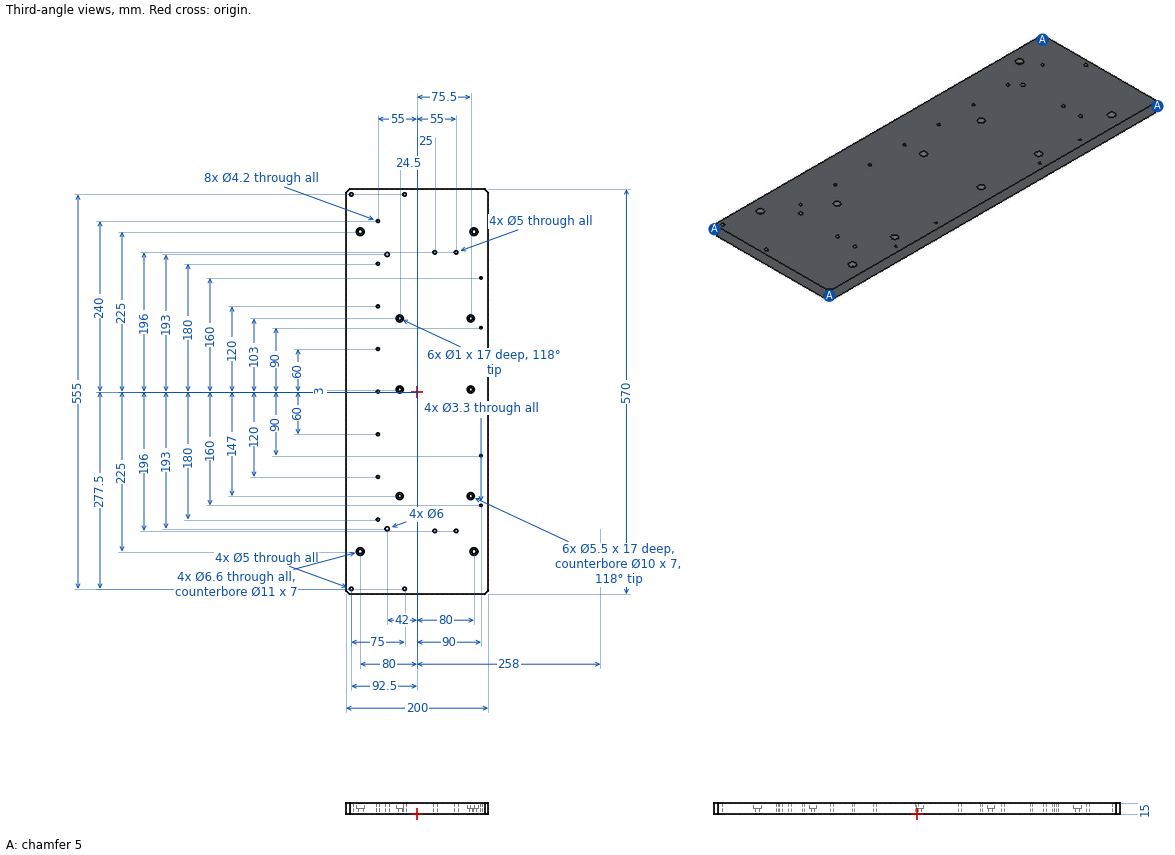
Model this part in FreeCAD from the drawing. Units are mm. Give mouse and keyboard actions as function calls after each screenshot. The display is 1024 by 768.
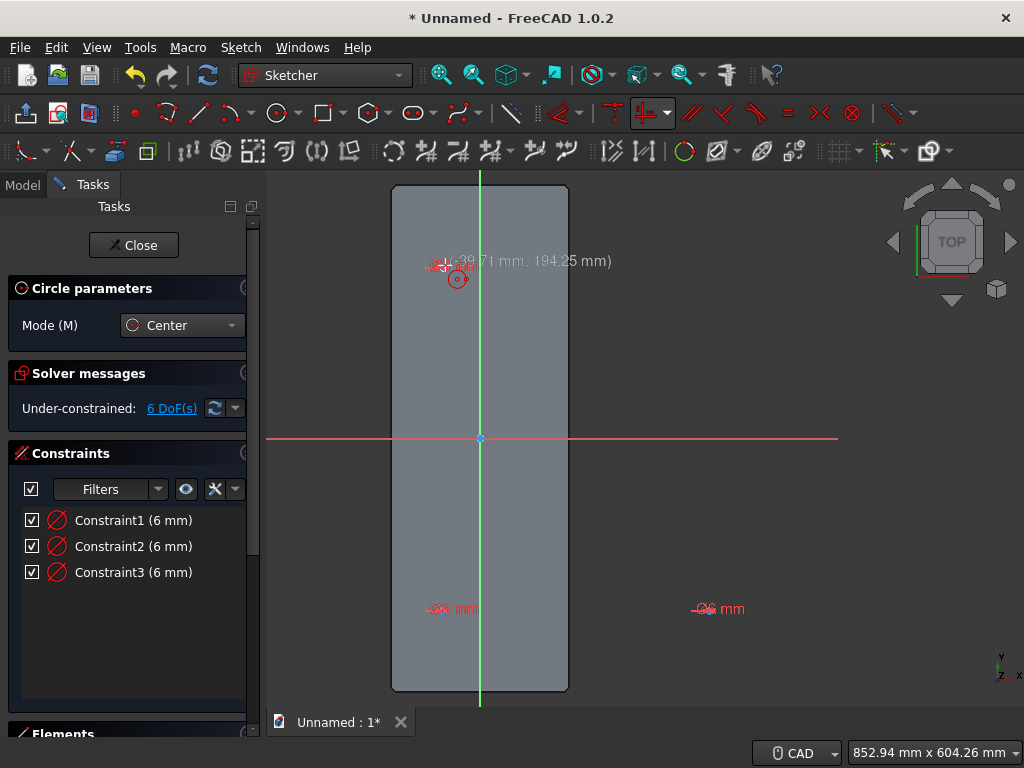
scroll(710, 267, up, 11)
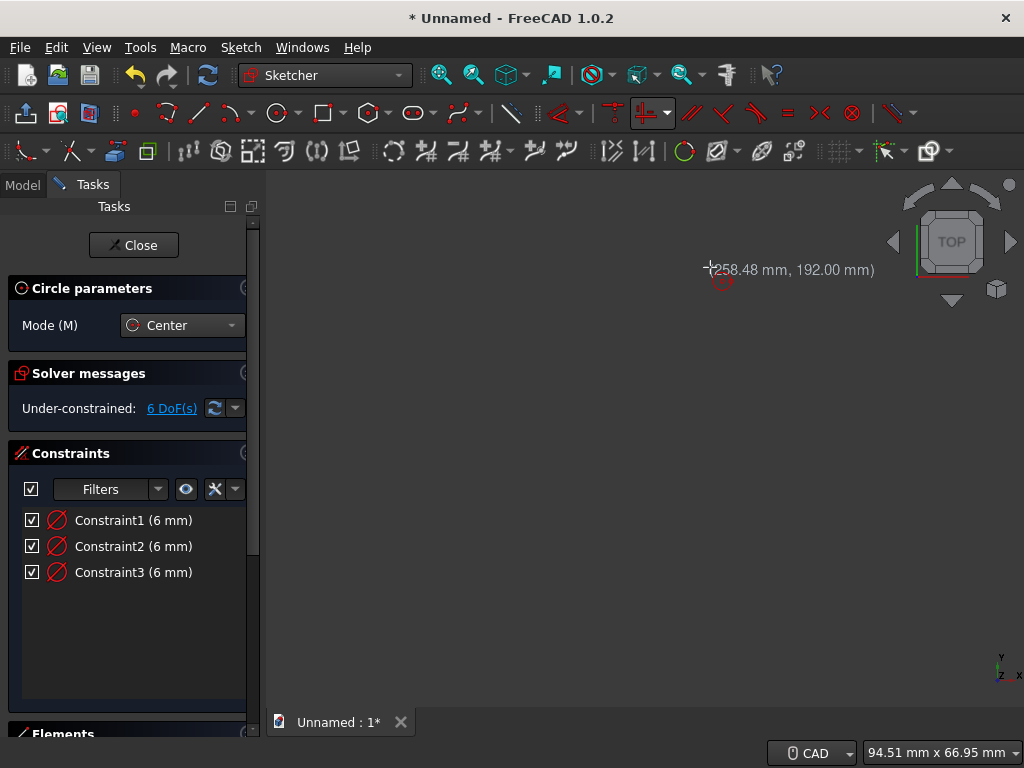
scroll(711, 267, down, 11)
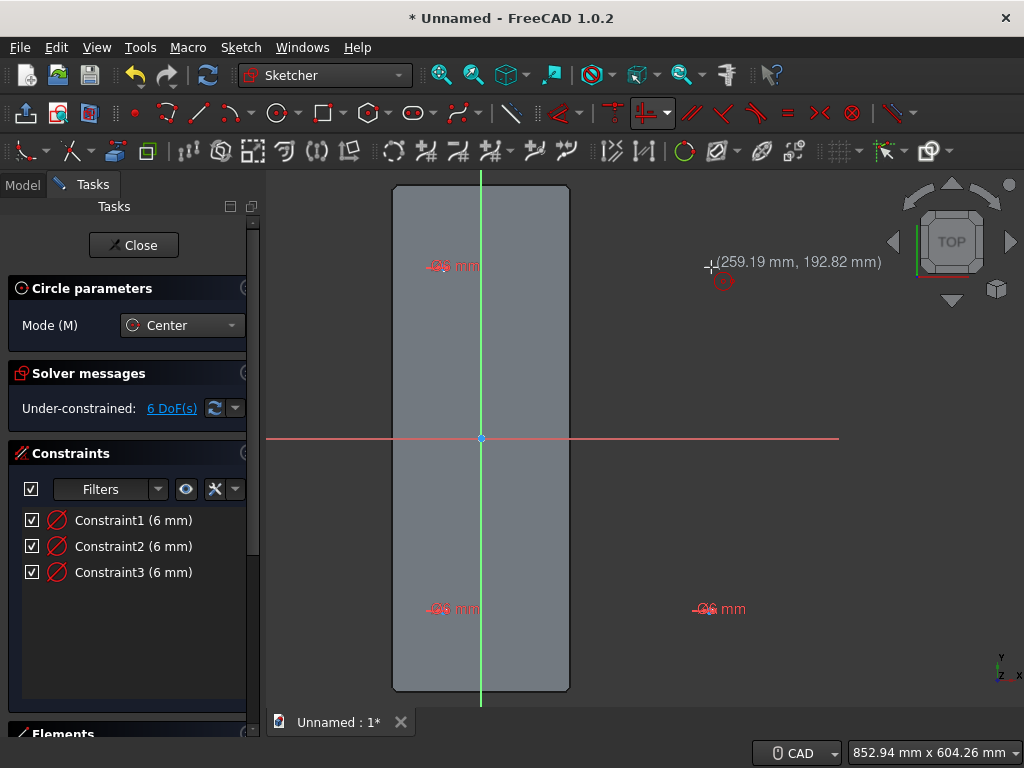
click(710, 267)
move(712, 265)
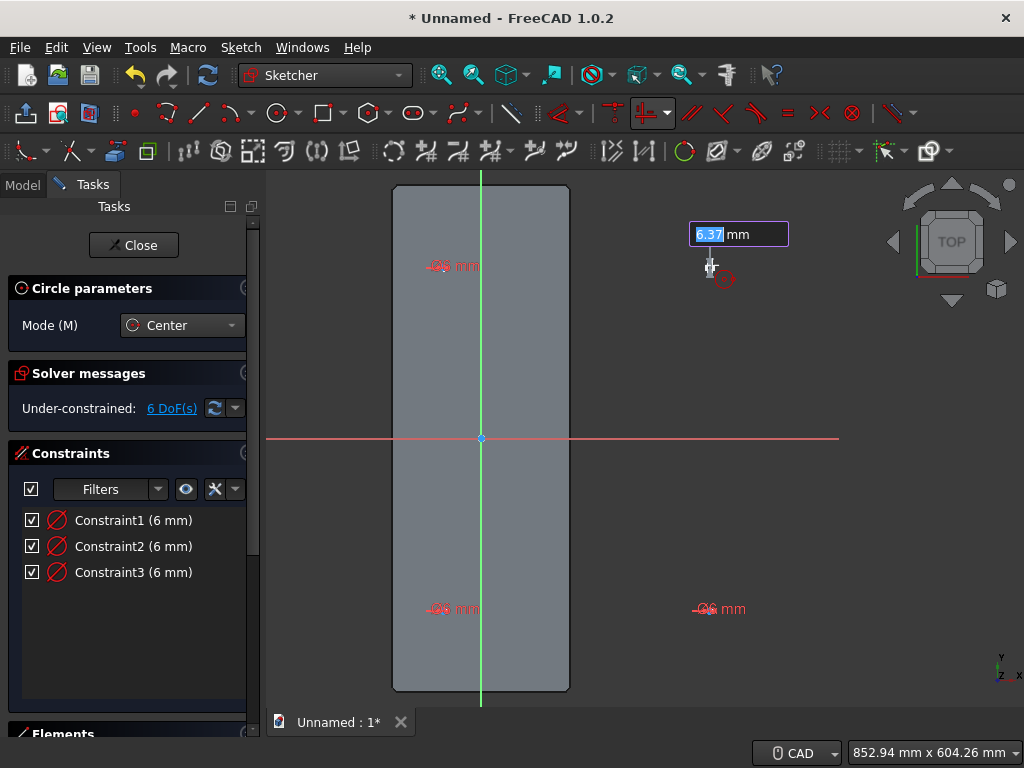
text(6)
key(Return)
key(Escape)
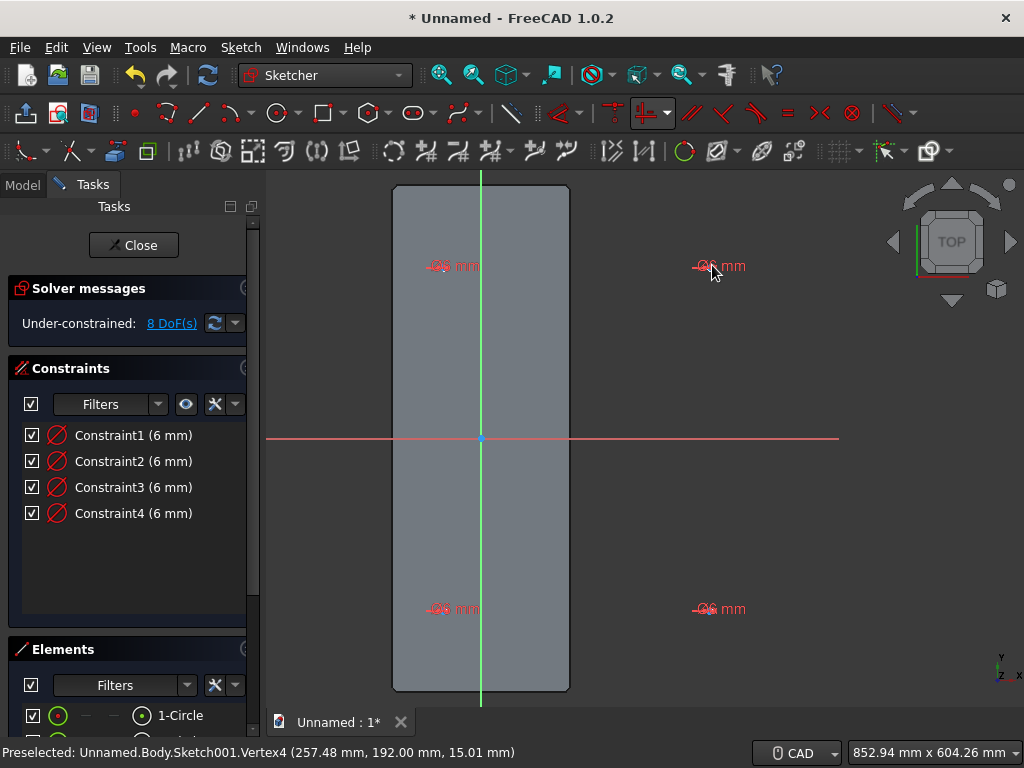
click(444, 611)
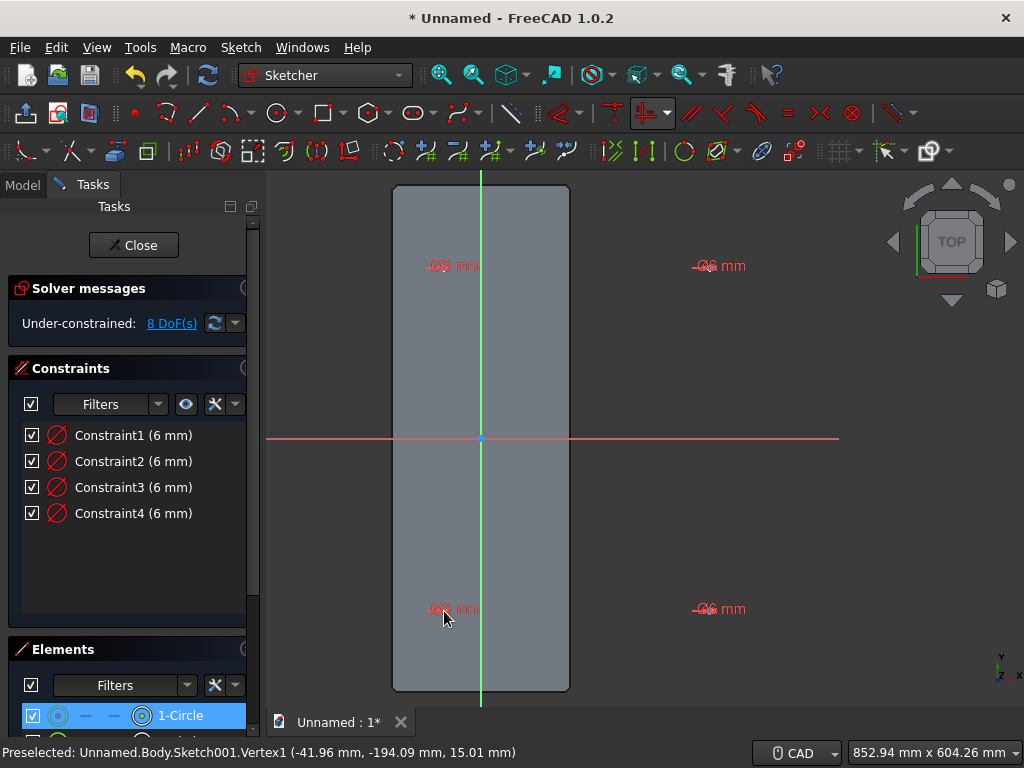
click(710, 611)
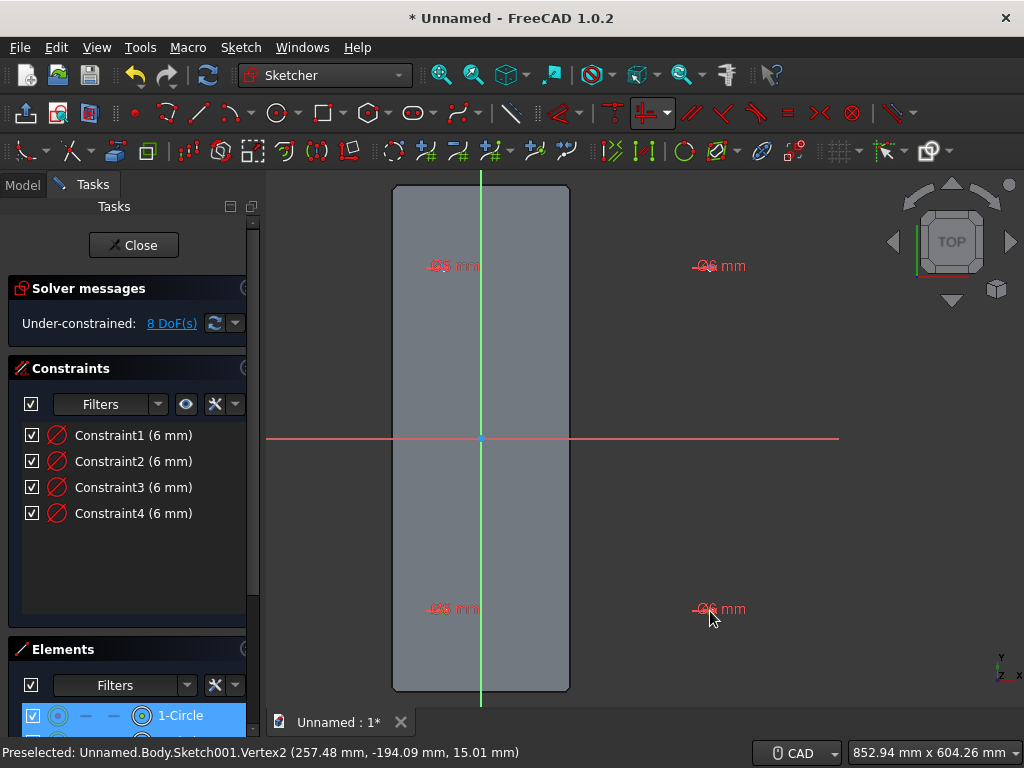
click(670, 114)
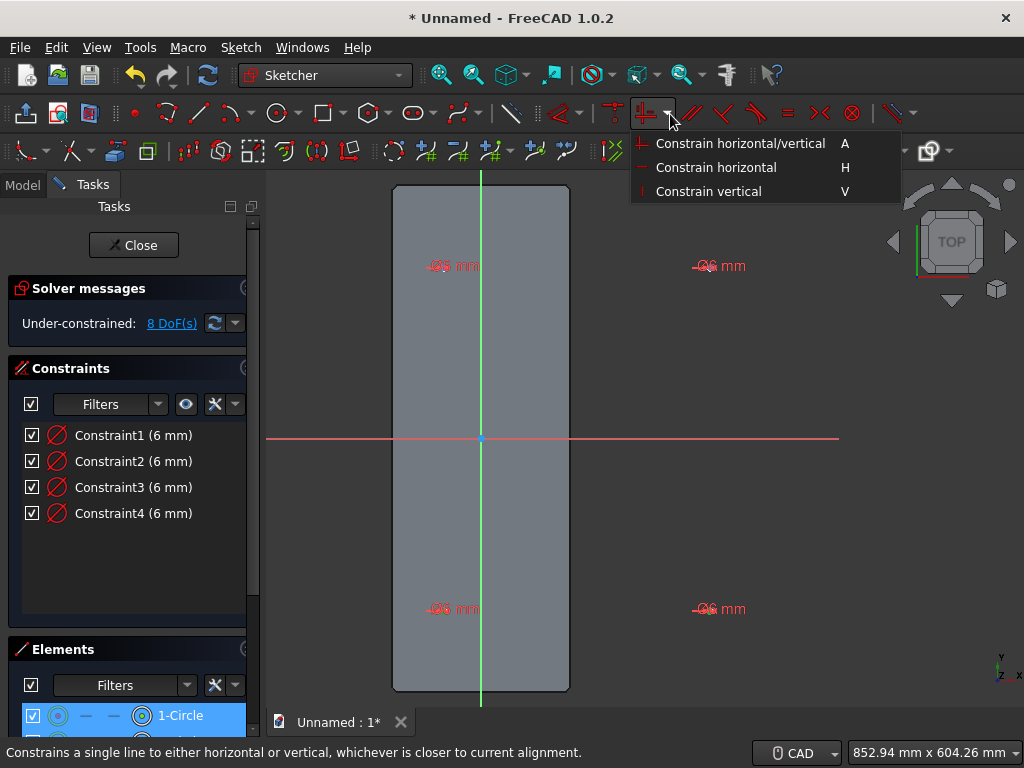
click(766, 167)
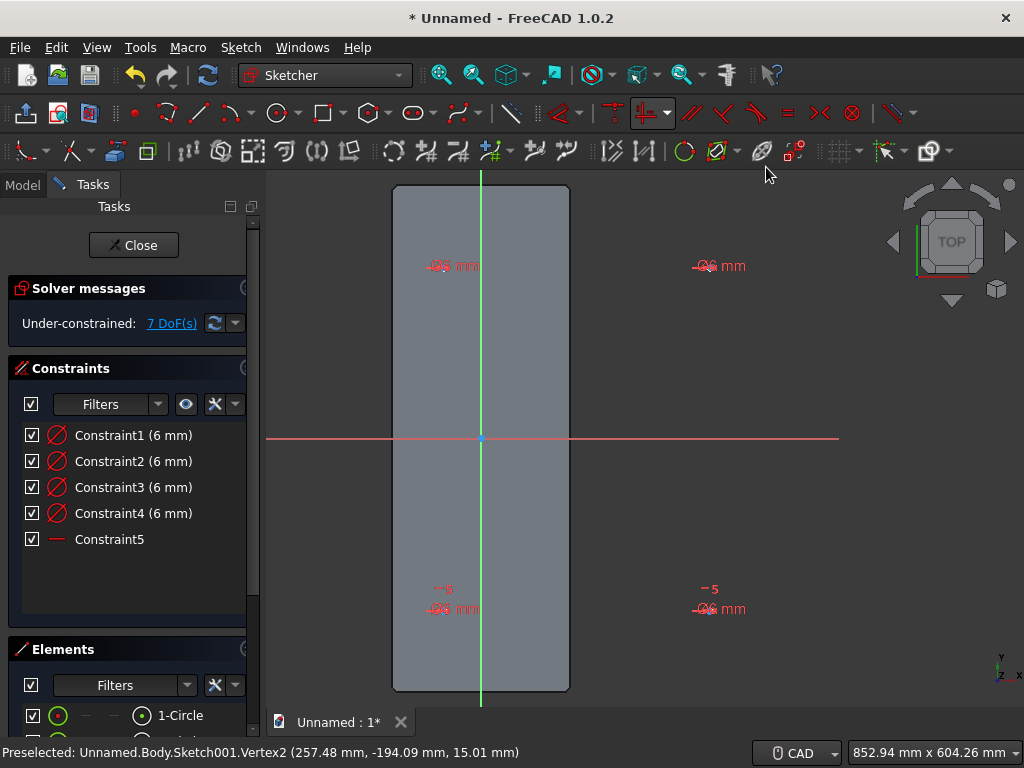
click(444, 611)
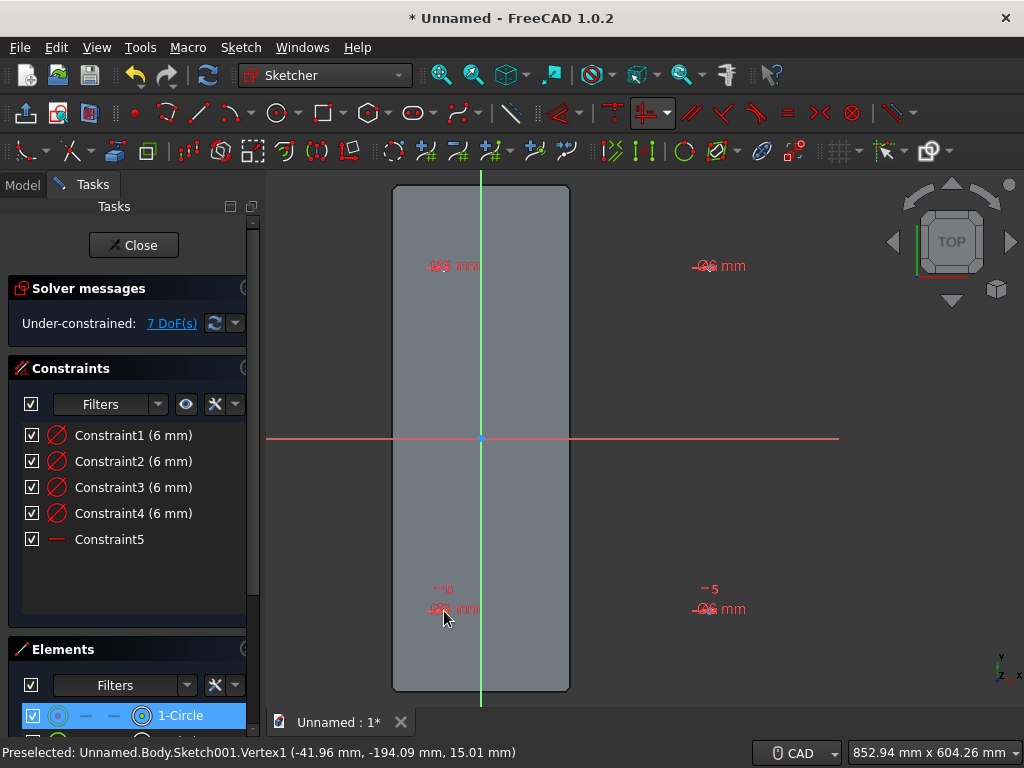
click(444, 268)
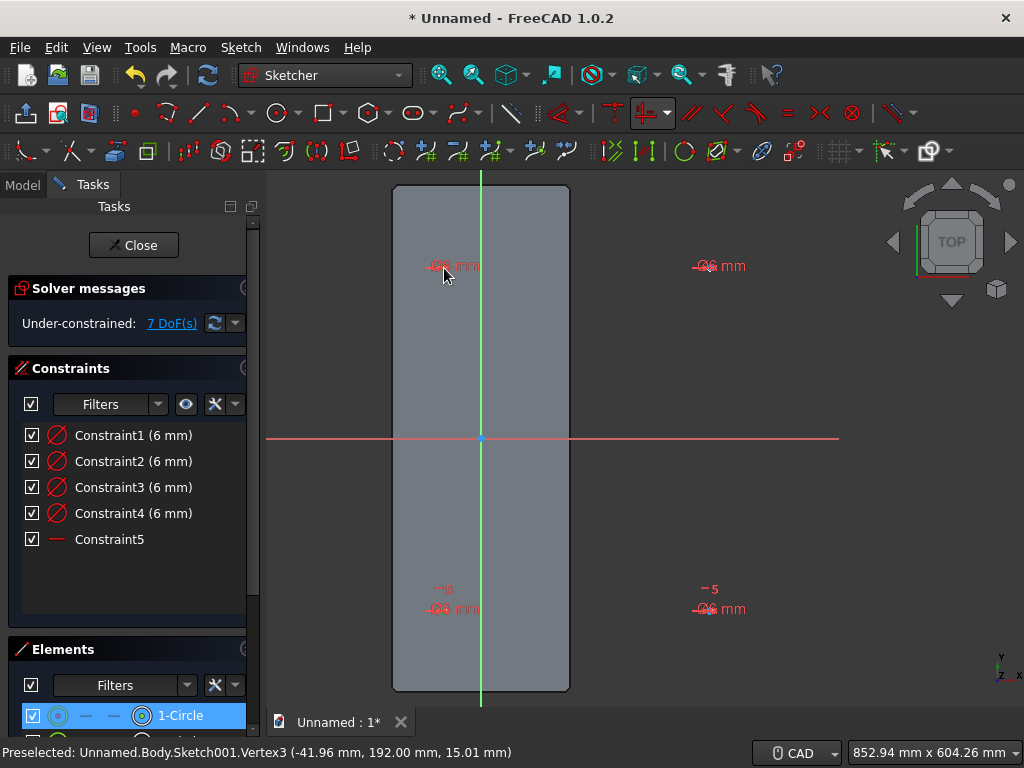
key(v)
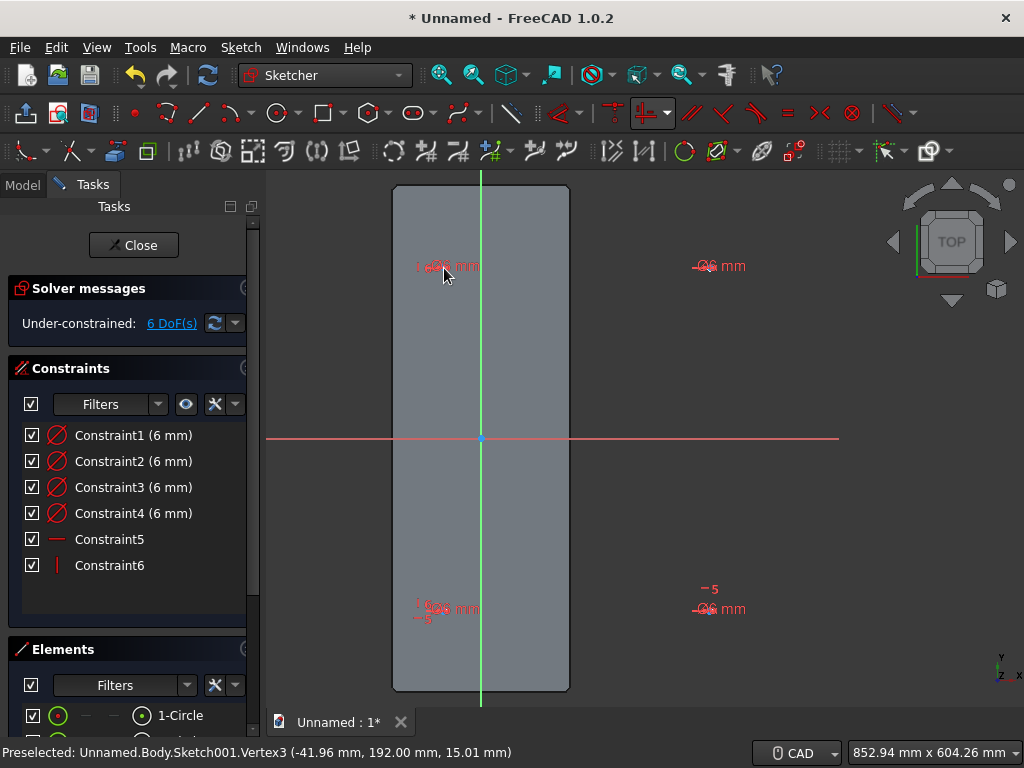
click(710, 611)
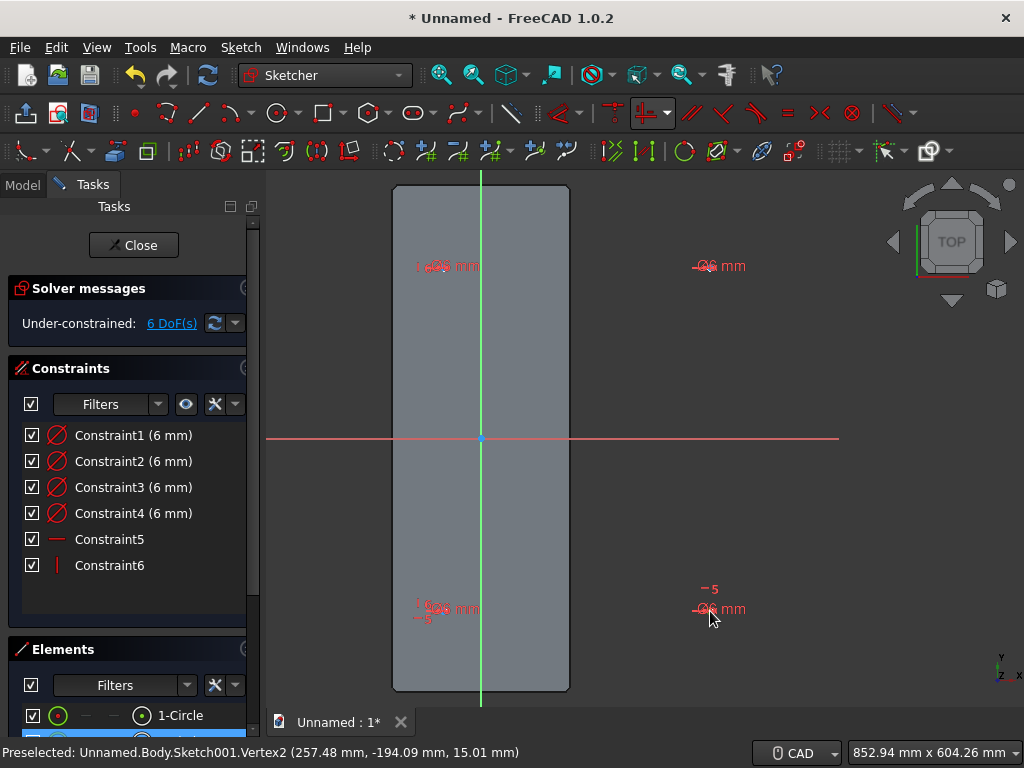
click(710, 268)